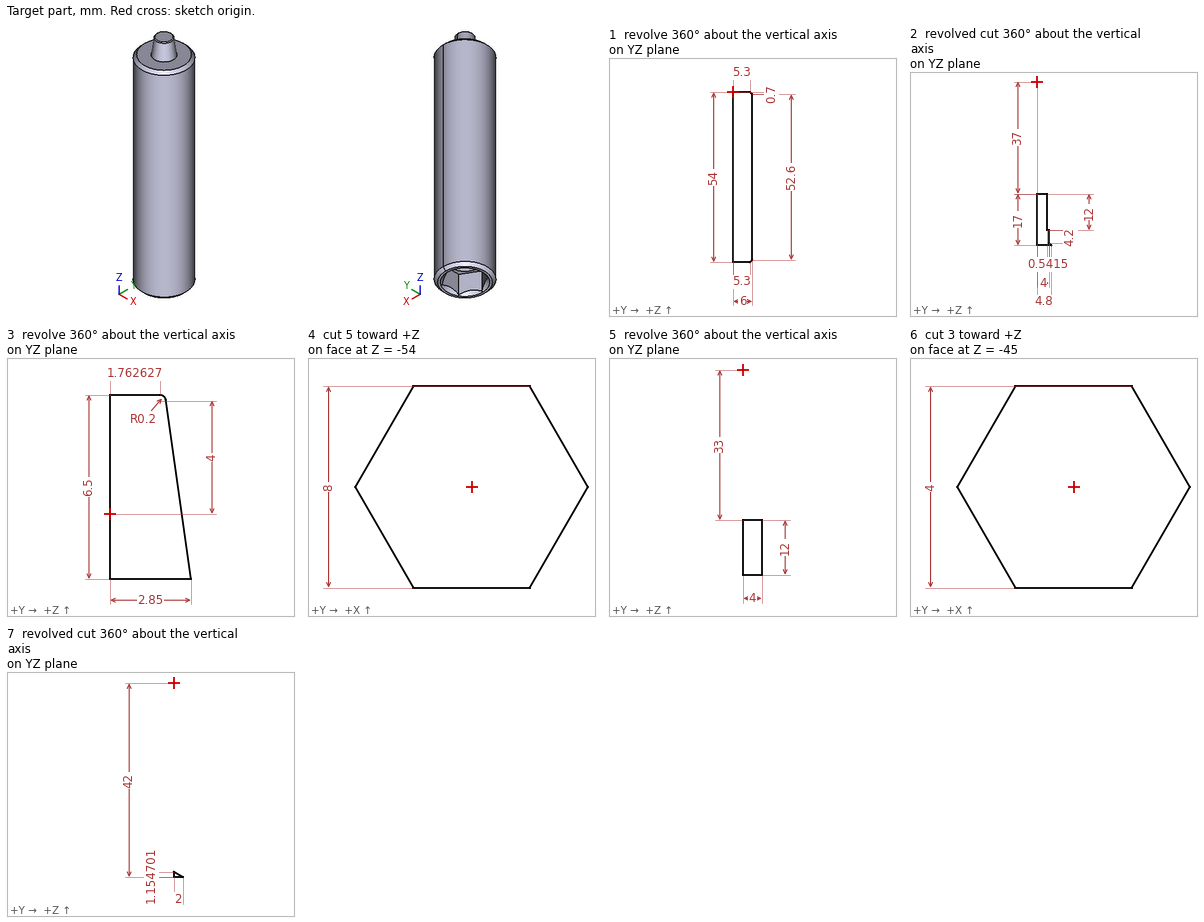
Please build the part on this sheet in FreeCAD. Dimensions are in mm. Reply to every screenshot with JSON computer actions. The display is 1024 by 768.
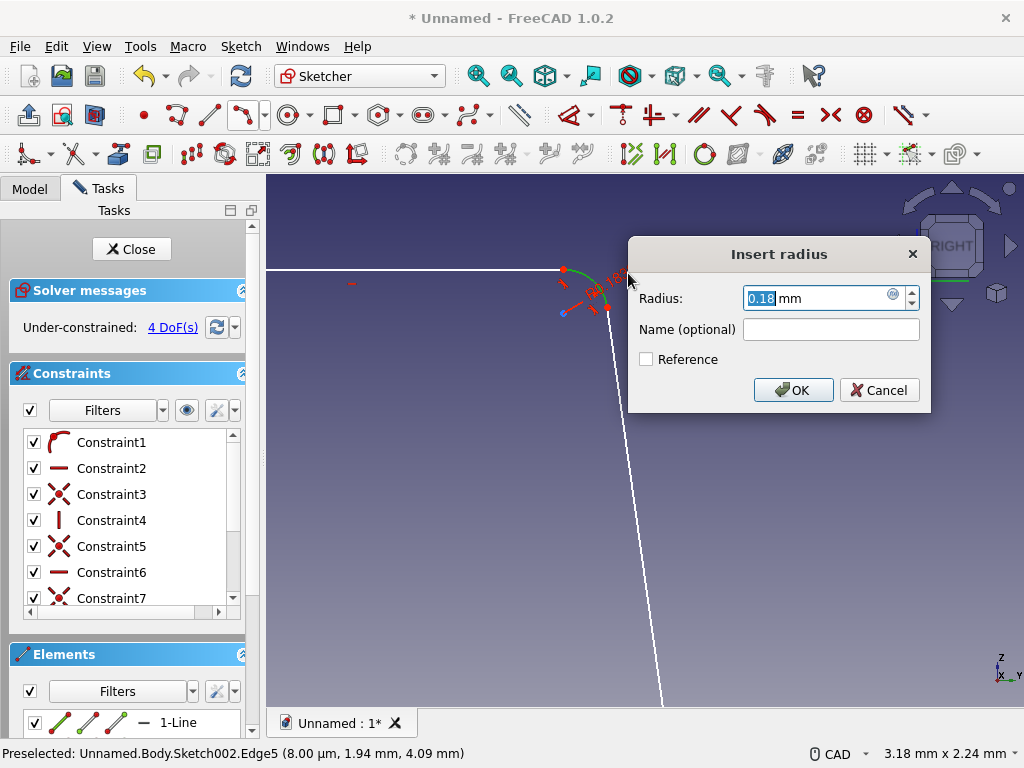
{"action": "type", "text": "0.2"}
{"action": "key", "text": "Return"}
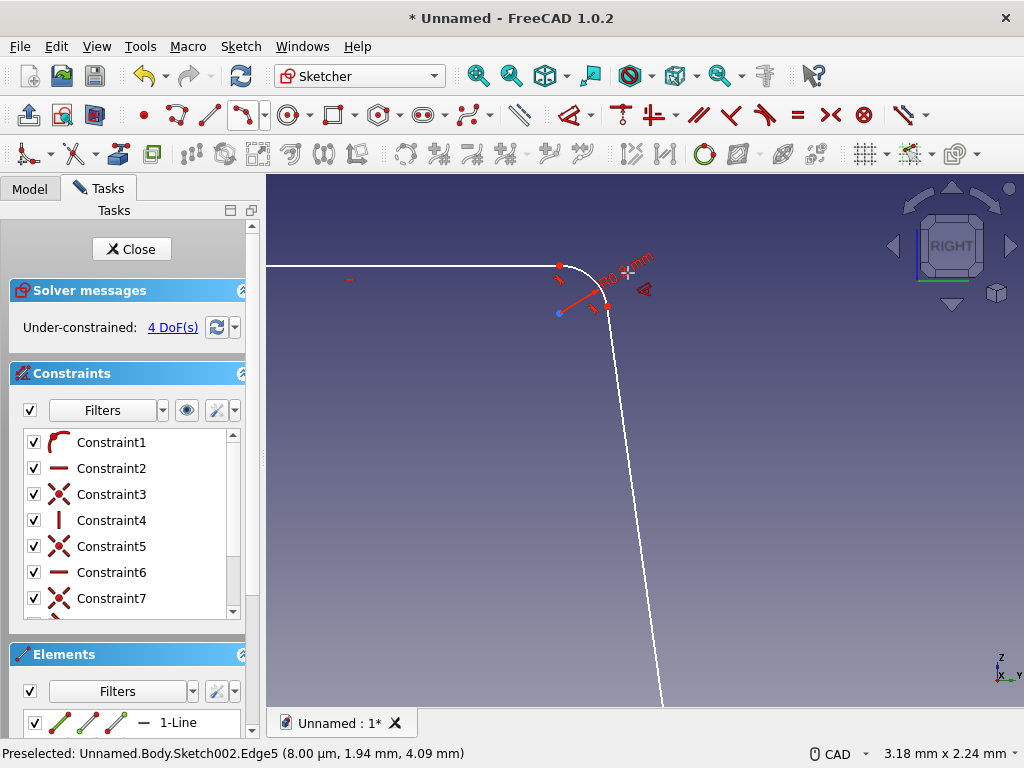
{"action": "scroll", "coordinate": [601, 288], "scroll_direction": "down", "scroll_amount": 8}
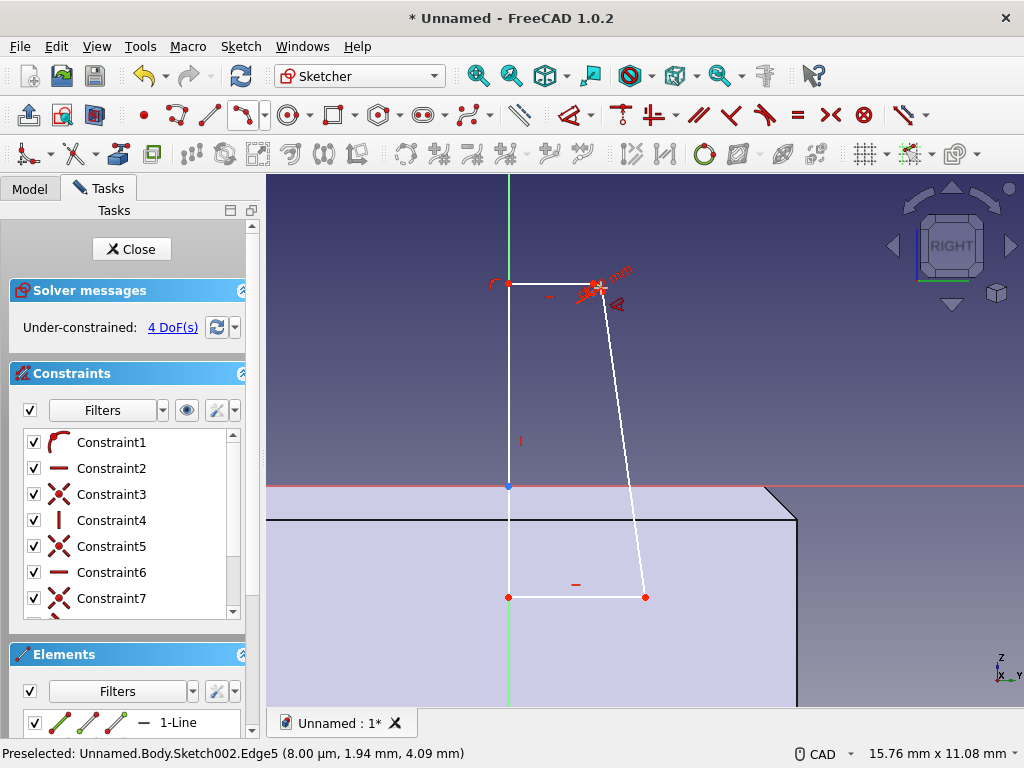
{"action": "scroll", "coordinate": [593, 293], "scroll_direction": "up", "scroll_amount": 2}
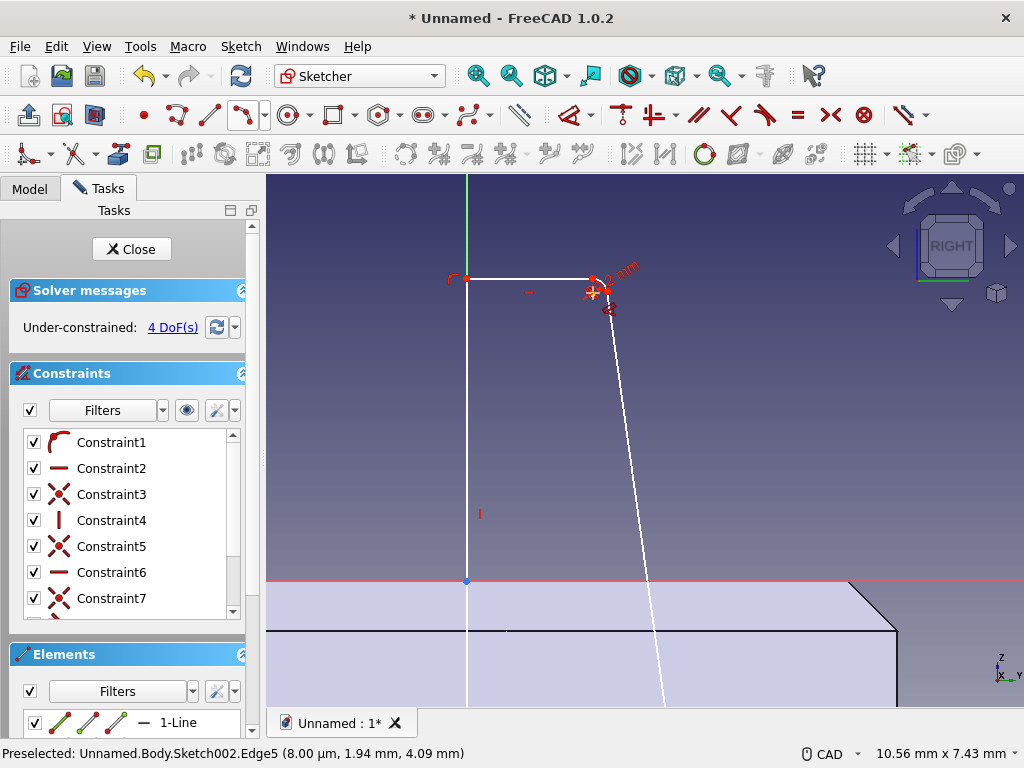
{"action": "left_click", "coordinate": [593, 293]}
{"action": "left_click", "coordinate": [433, 437]}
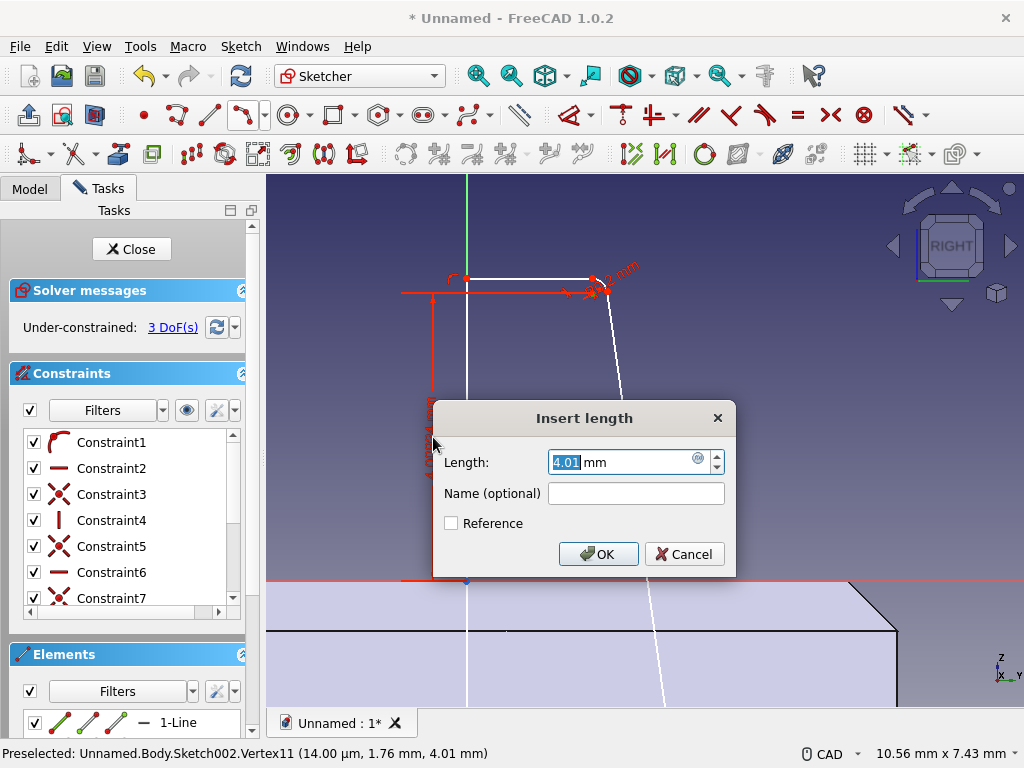
{"action": "type", "text": "4"}
{"action": "key", "text": "Return"}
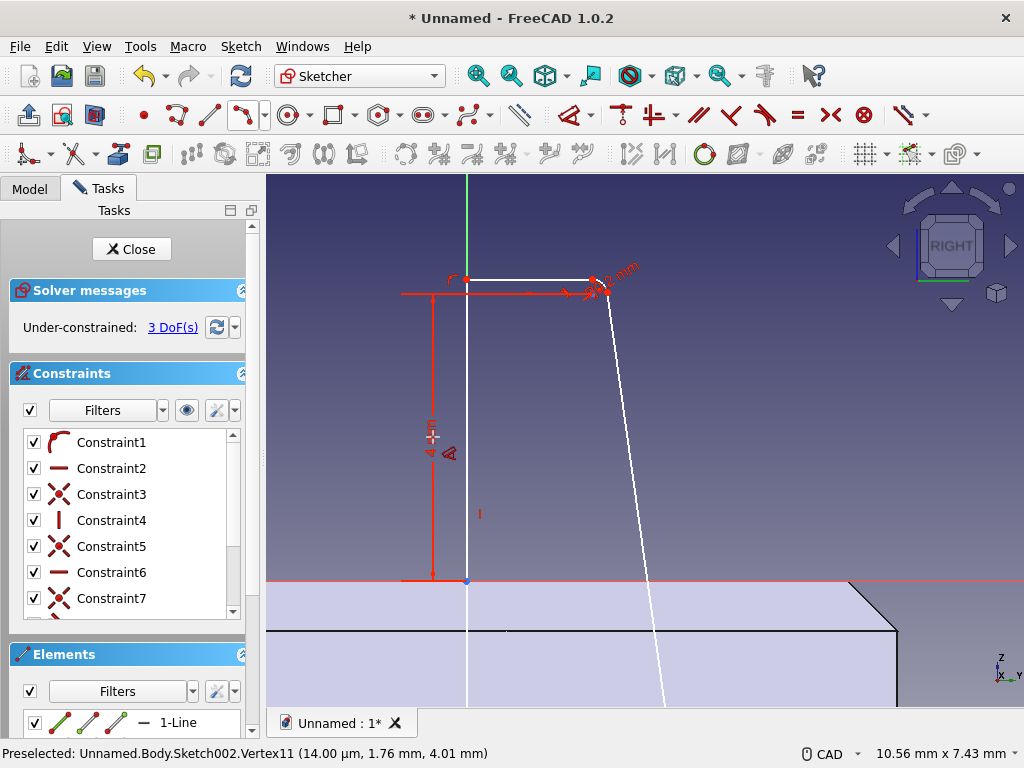
{"action": "left_click", "coordinate": [467, 420]}
{"action": "left_click", "coordinate": [433, 479]}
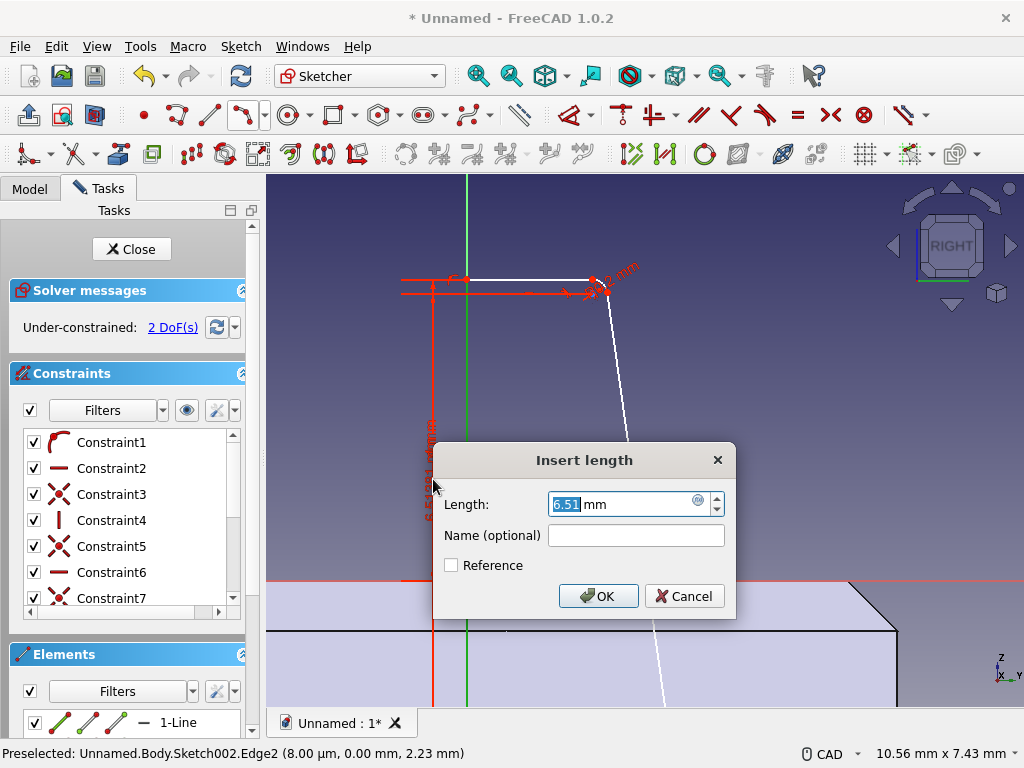
{"action": "type", "text": "6.5"}
{"action": "key", "text": "Return"}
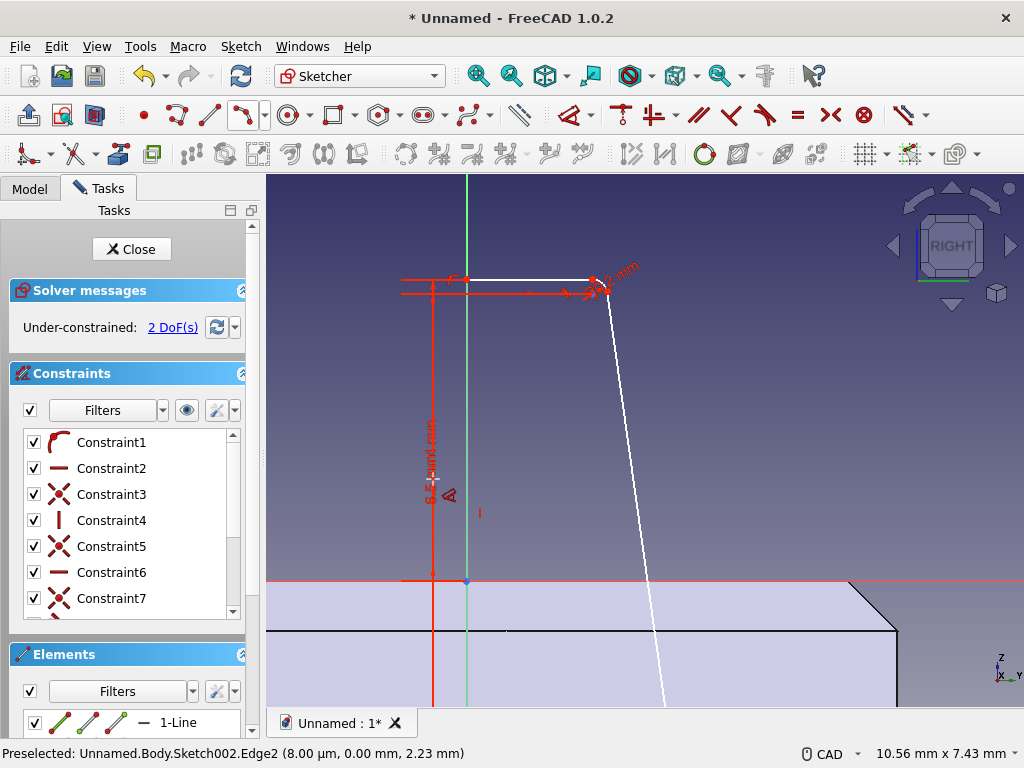
{"action": "scroll", "coordinate": [592, 293], "scroll_direction": "down", "scroll_amount": 2}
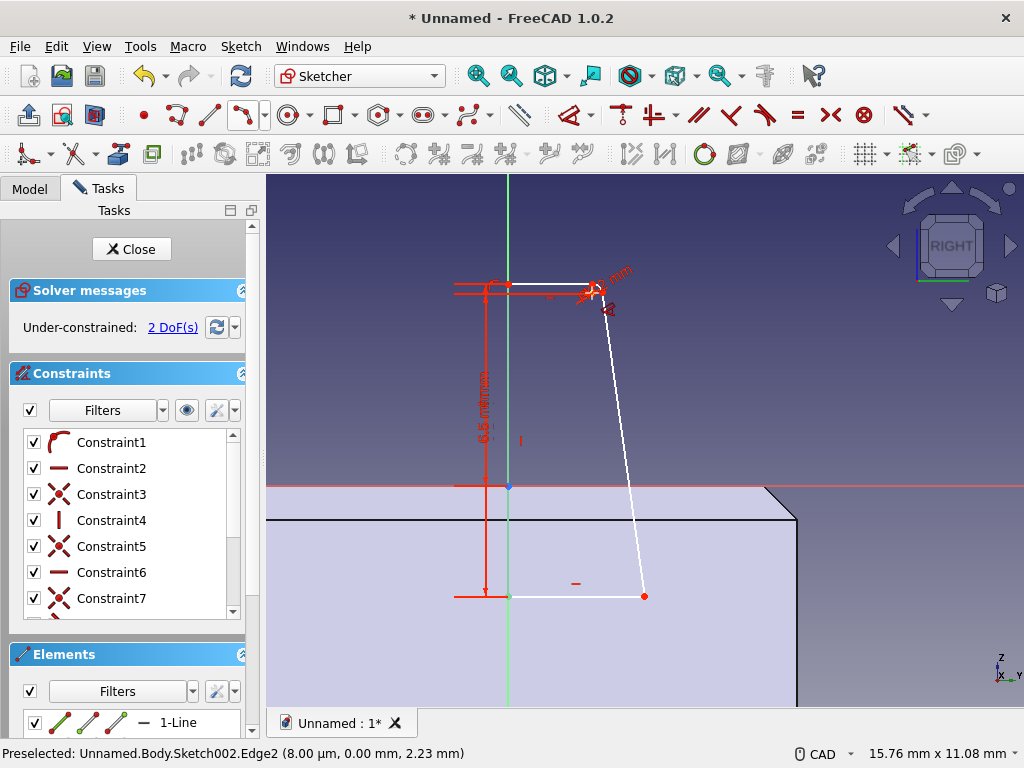
{"action": "left_click", "coordinate": [549, 597]}
{"action": "left_click", "coordinate": [577, 631]}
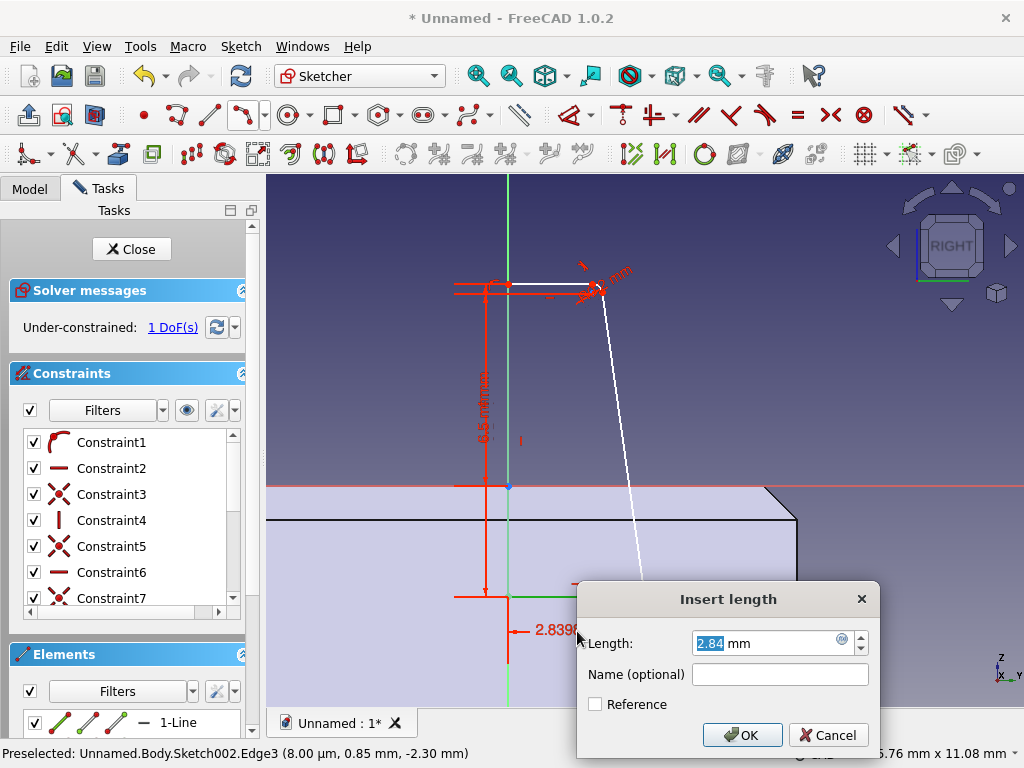
{"action": "type", "text": "2.85"}
{"action": "key", "text": "Return"}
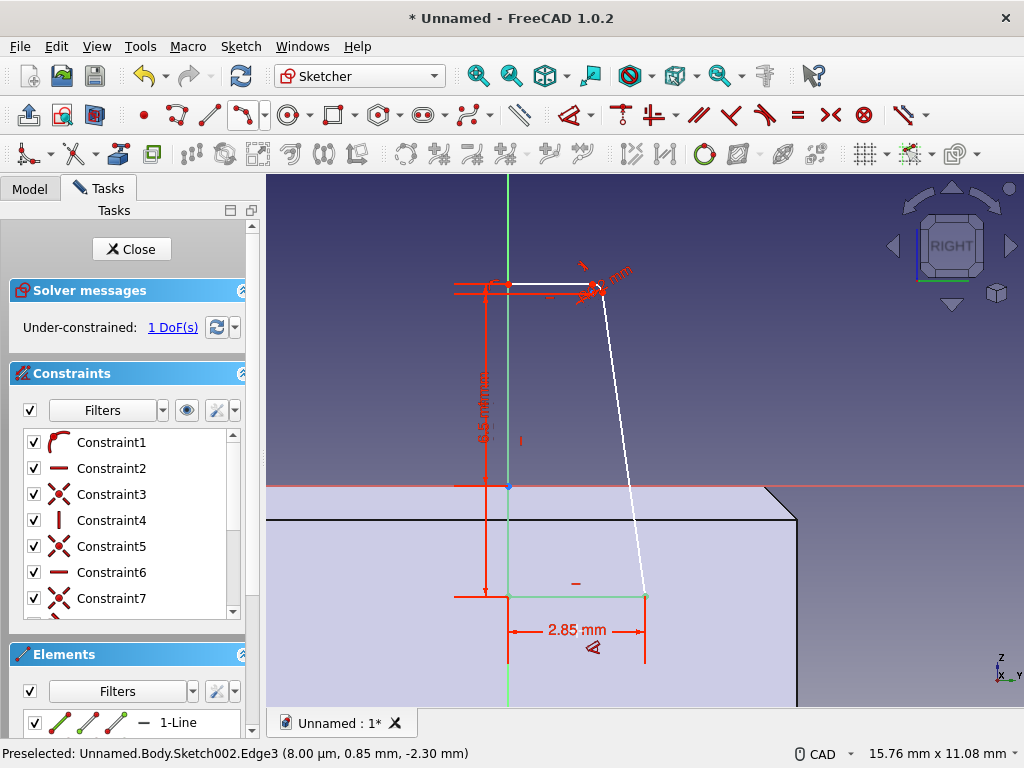
{"action": "left_click", "coordinate": [567, 284]}
{"action": "left_click", "coordinate": [550, 250]}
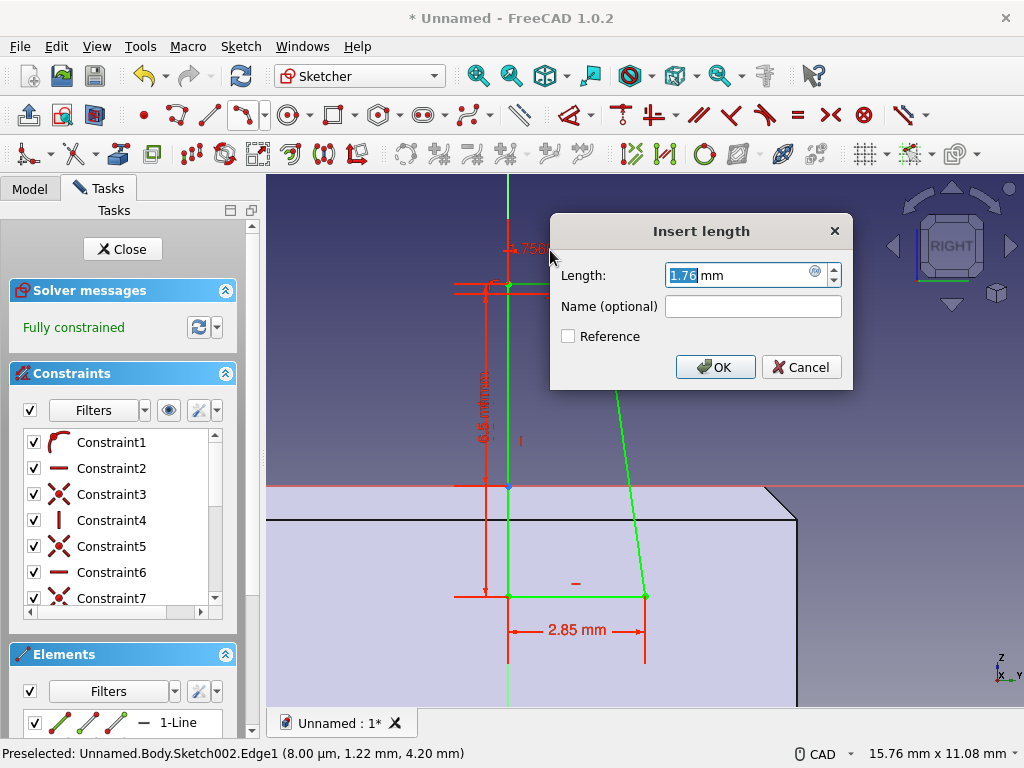
{"action": "type", "text": "1.762627"}
{"action": "key", "text": "Return"}
{"action": "key", "text": "Escape"}